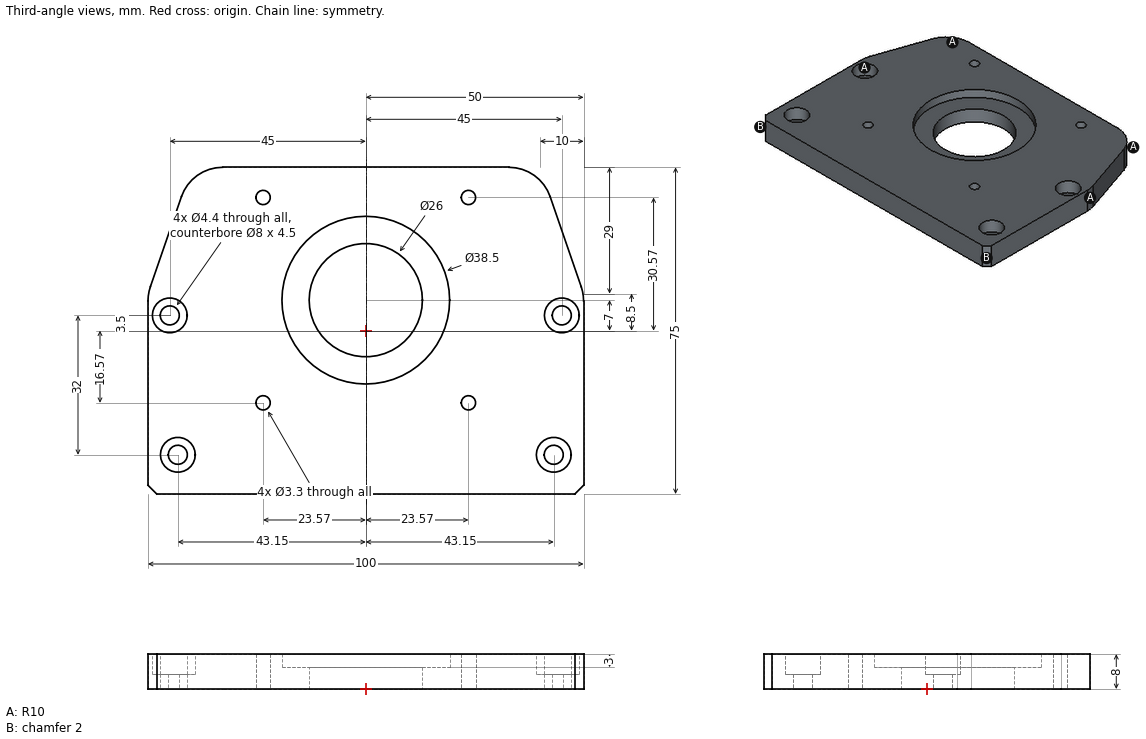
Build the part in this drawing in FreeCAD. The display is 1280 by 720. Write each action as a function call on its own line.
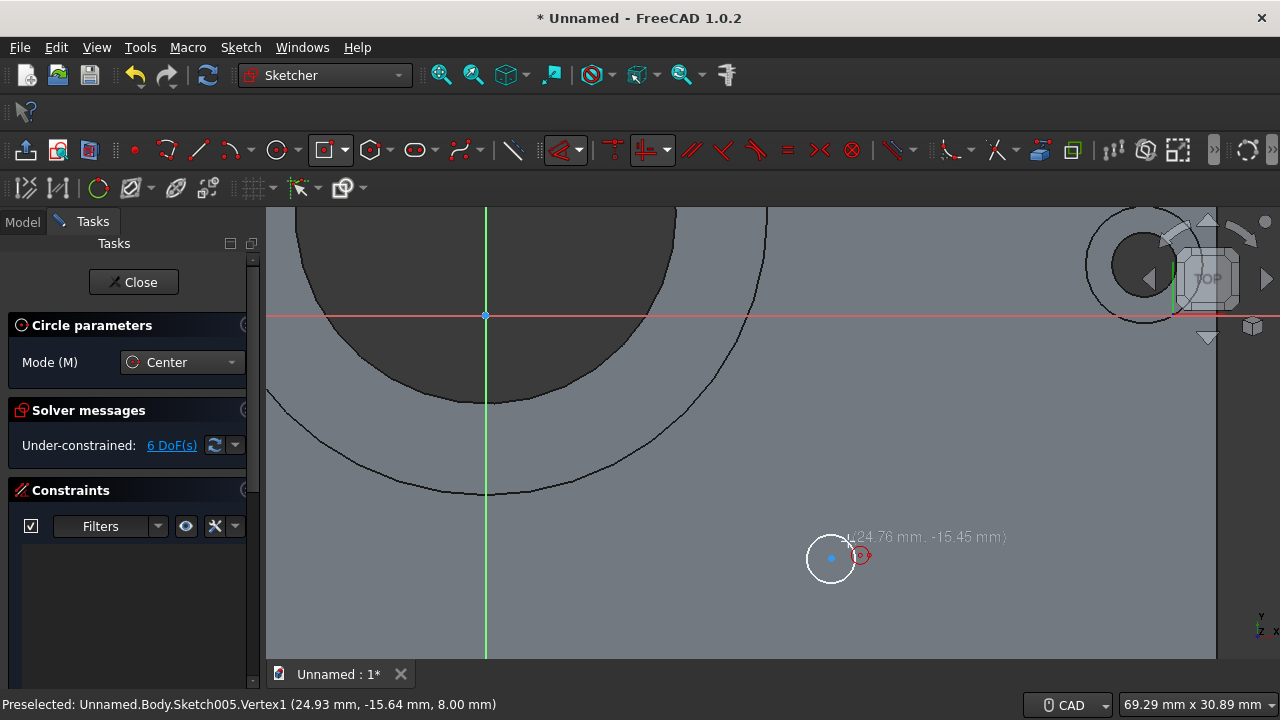
scroll(832, 561, down, 5)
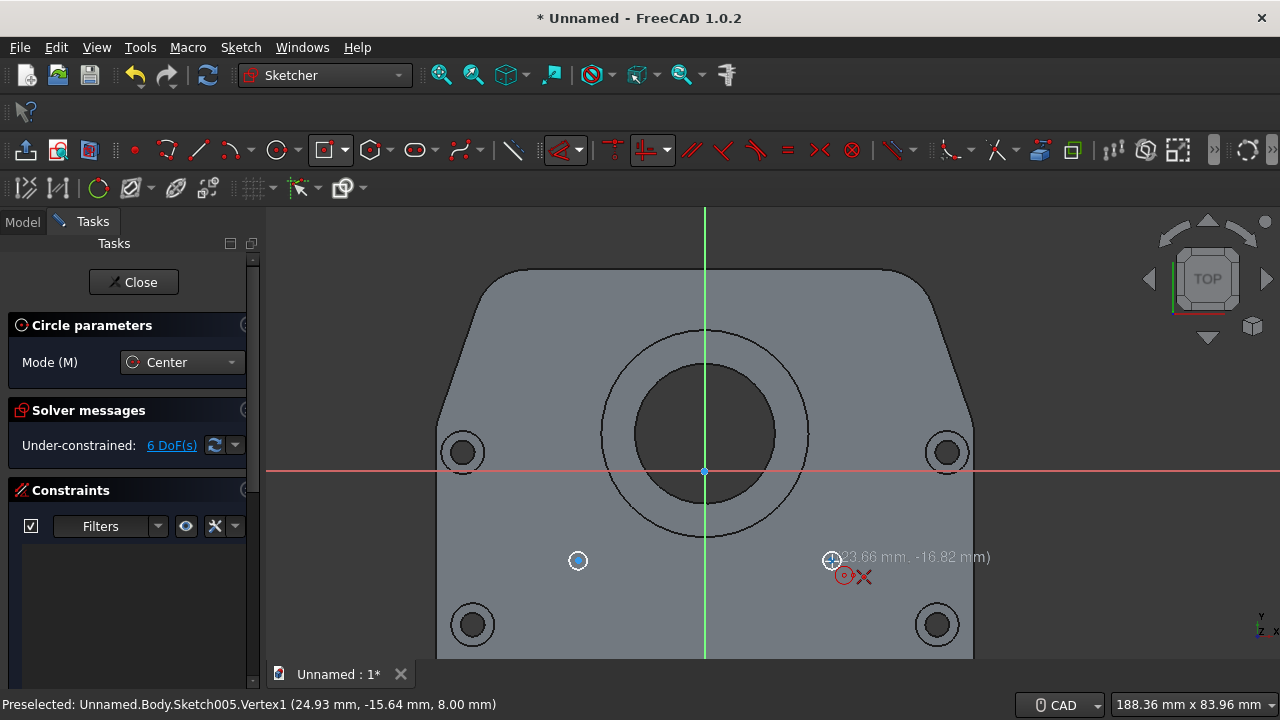
scroll(832, 307, up, 5)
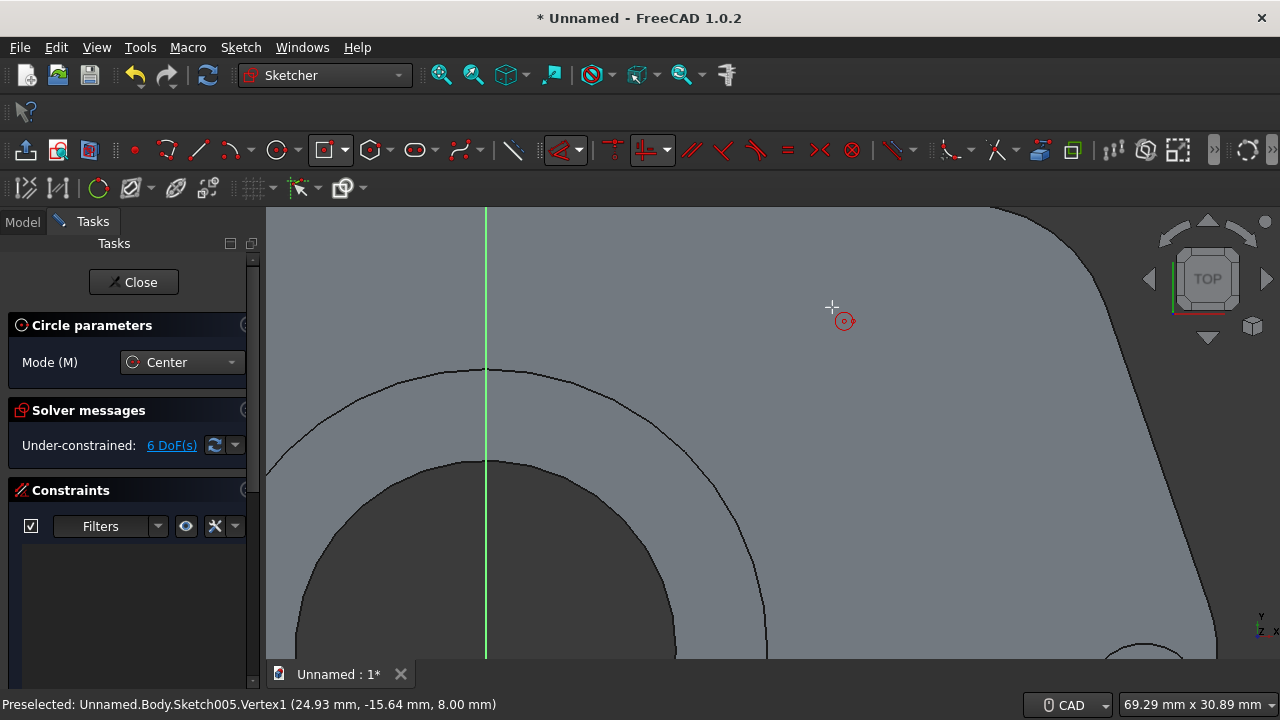
click(831, 306)
click(848, 289)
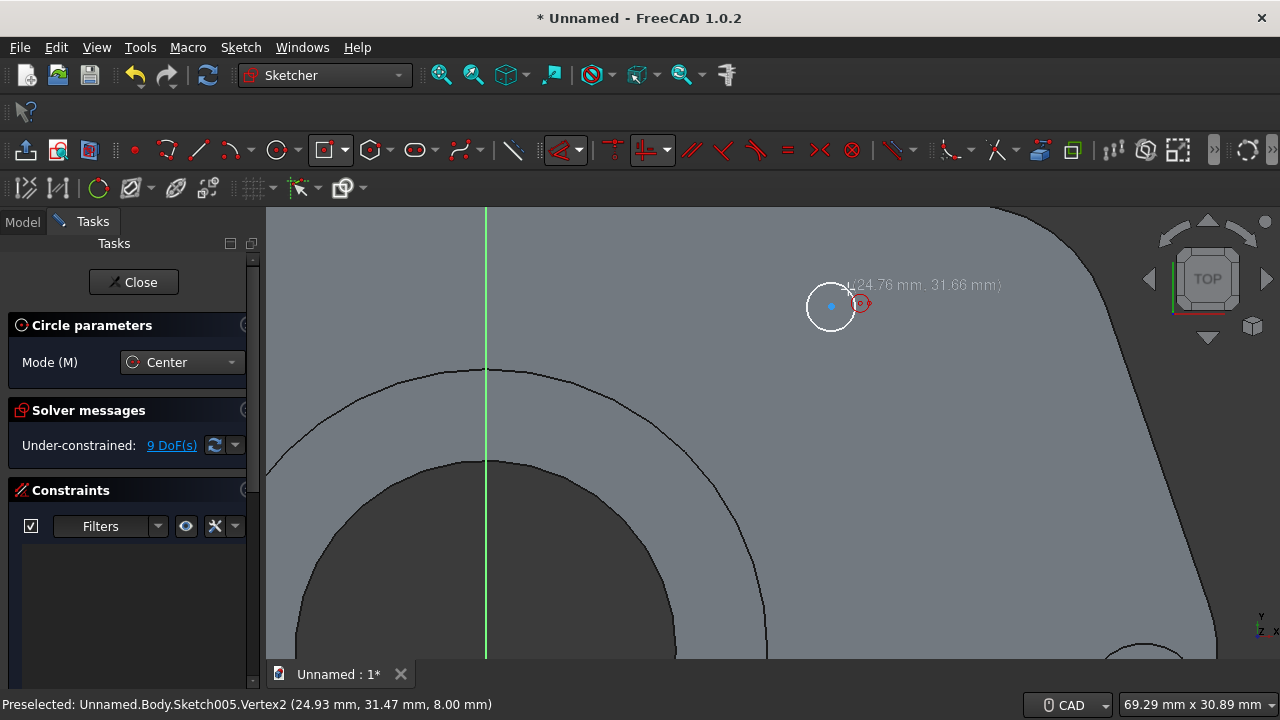
scroll(832, 306, down, 5)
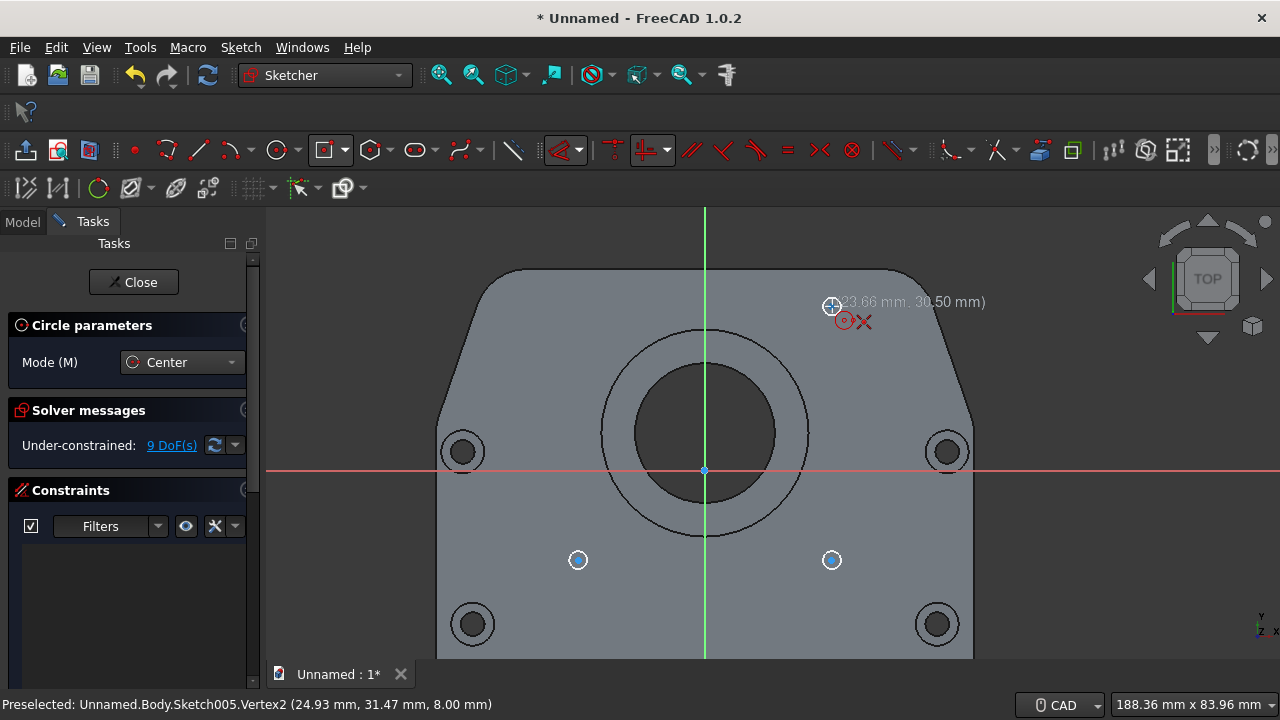
scroll(578, 306, up, 5)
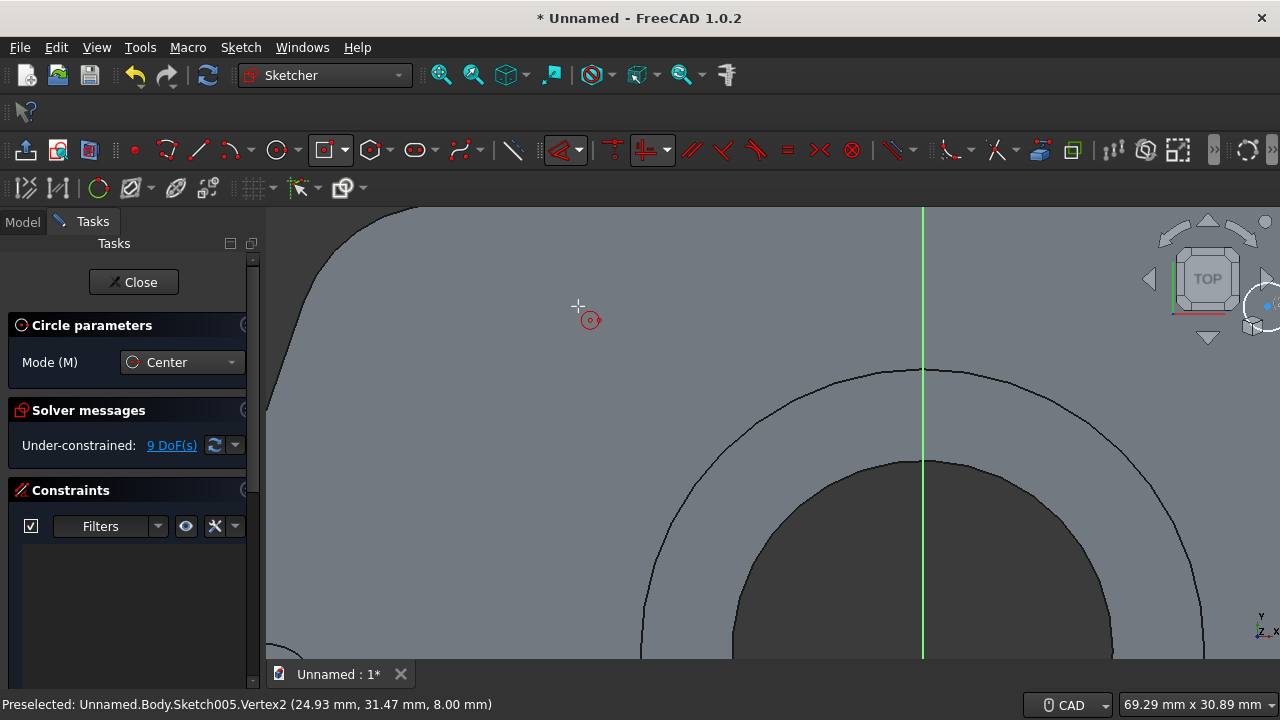
click(578, 306)
click(595, 289)
key(Escape)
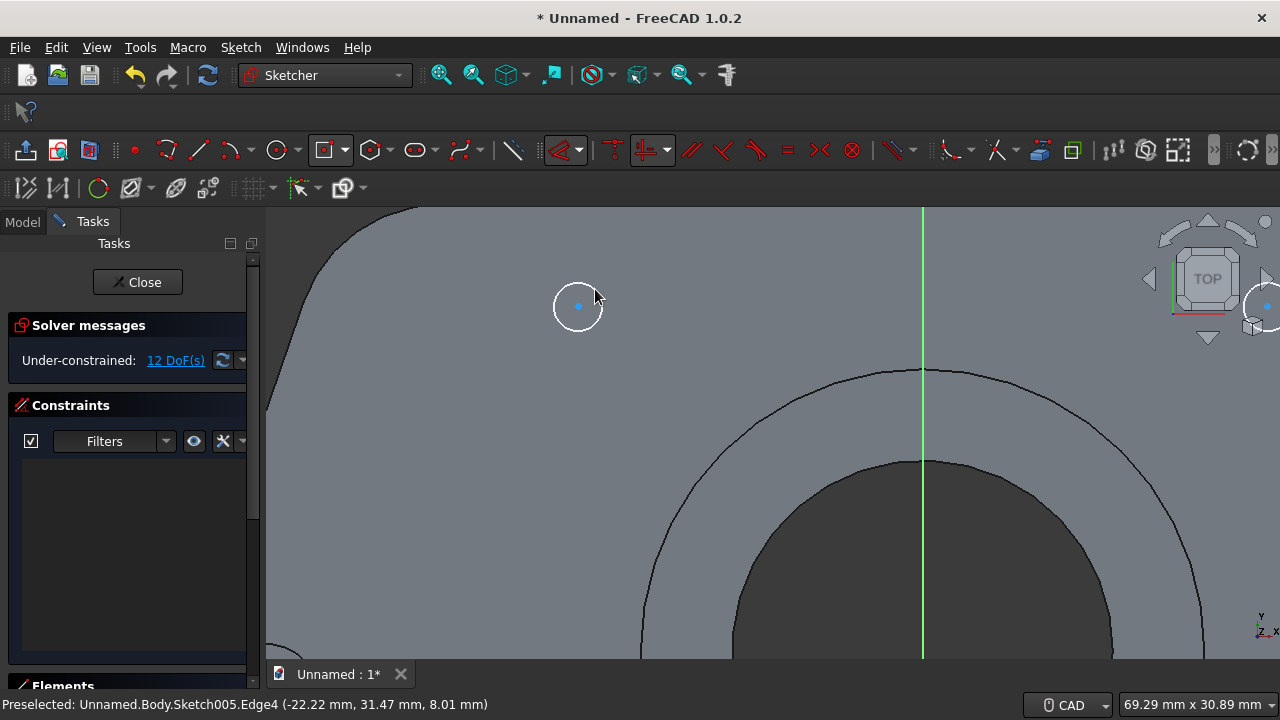
scroll(578, 306, down, 5)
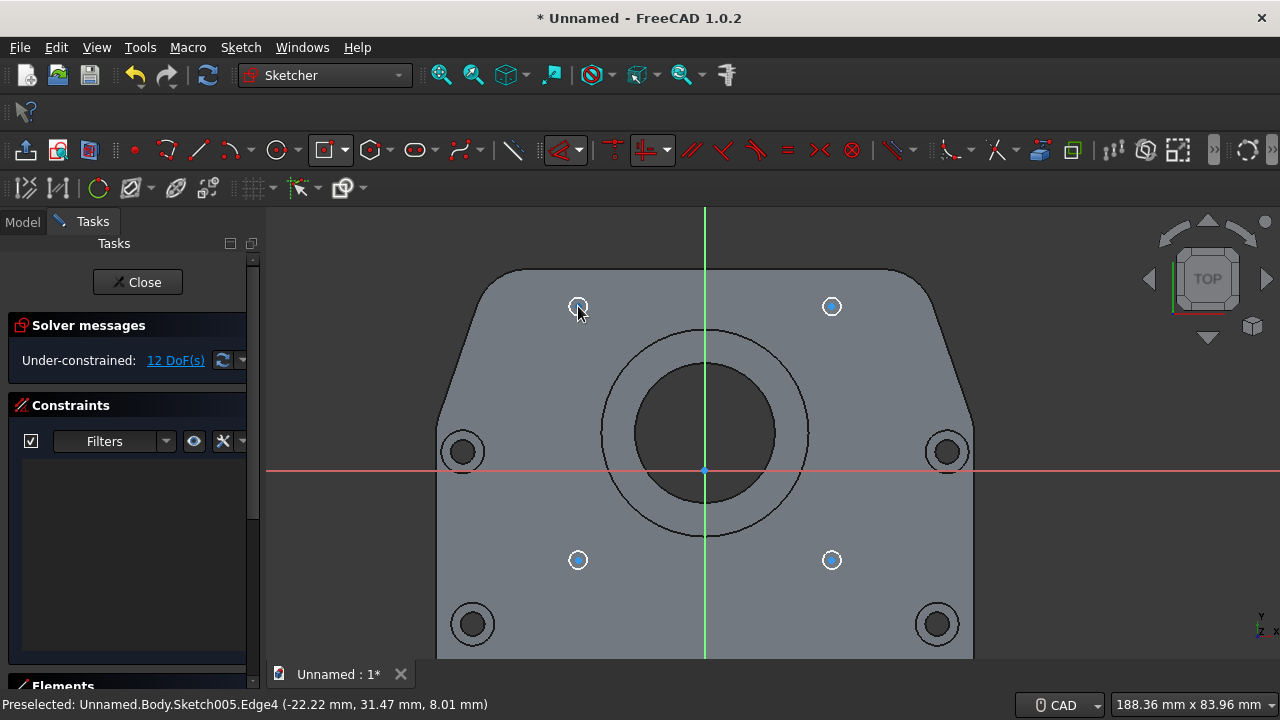
scroll(584, 554, up, 3)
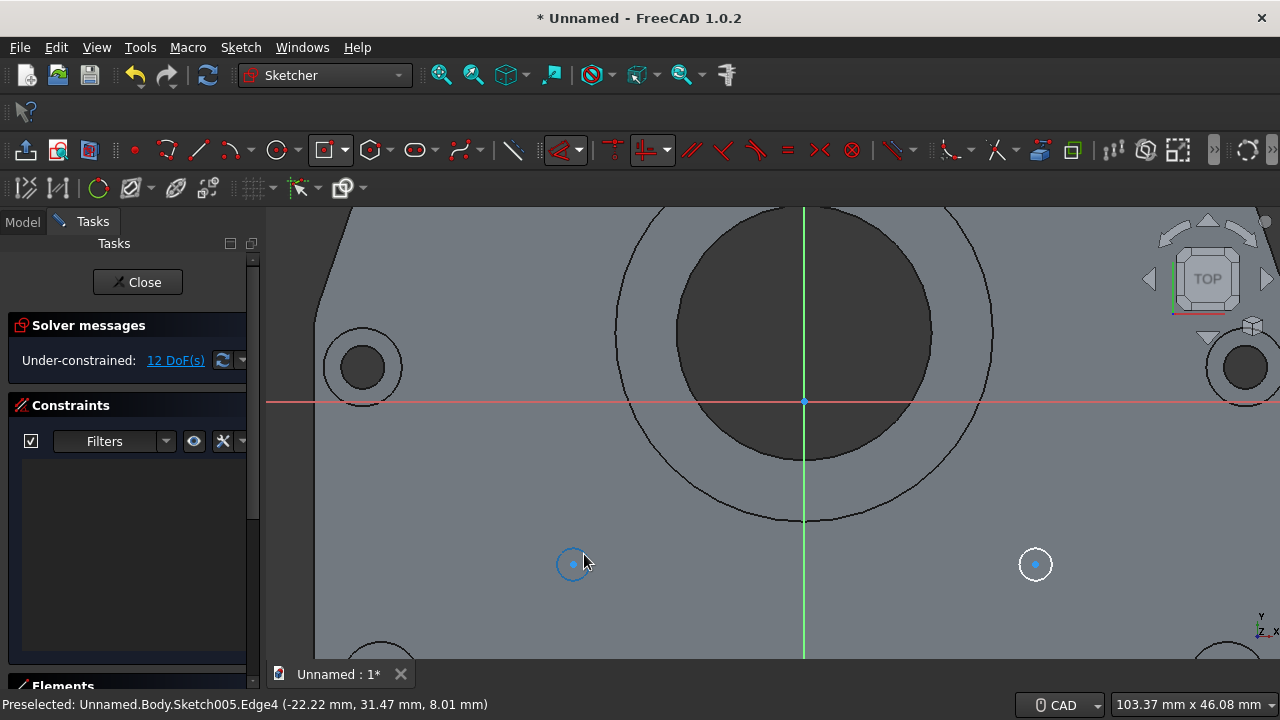
click(585, 553)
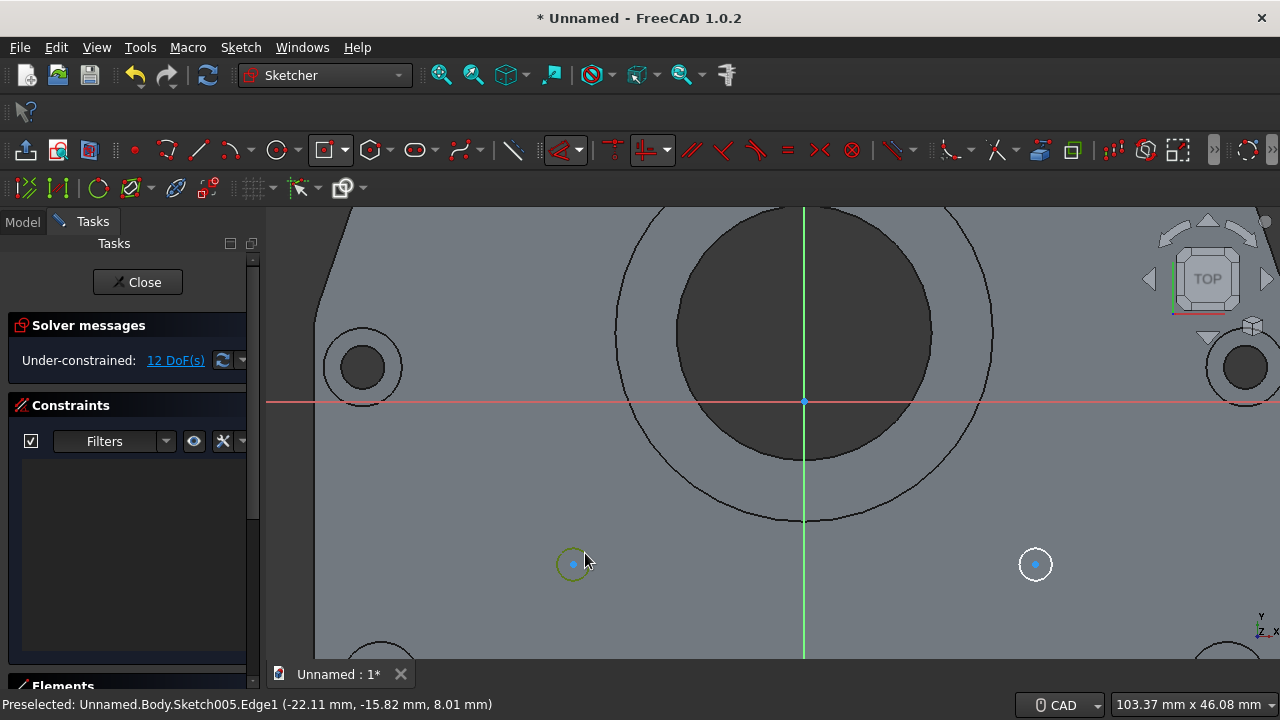
click(1047, 553)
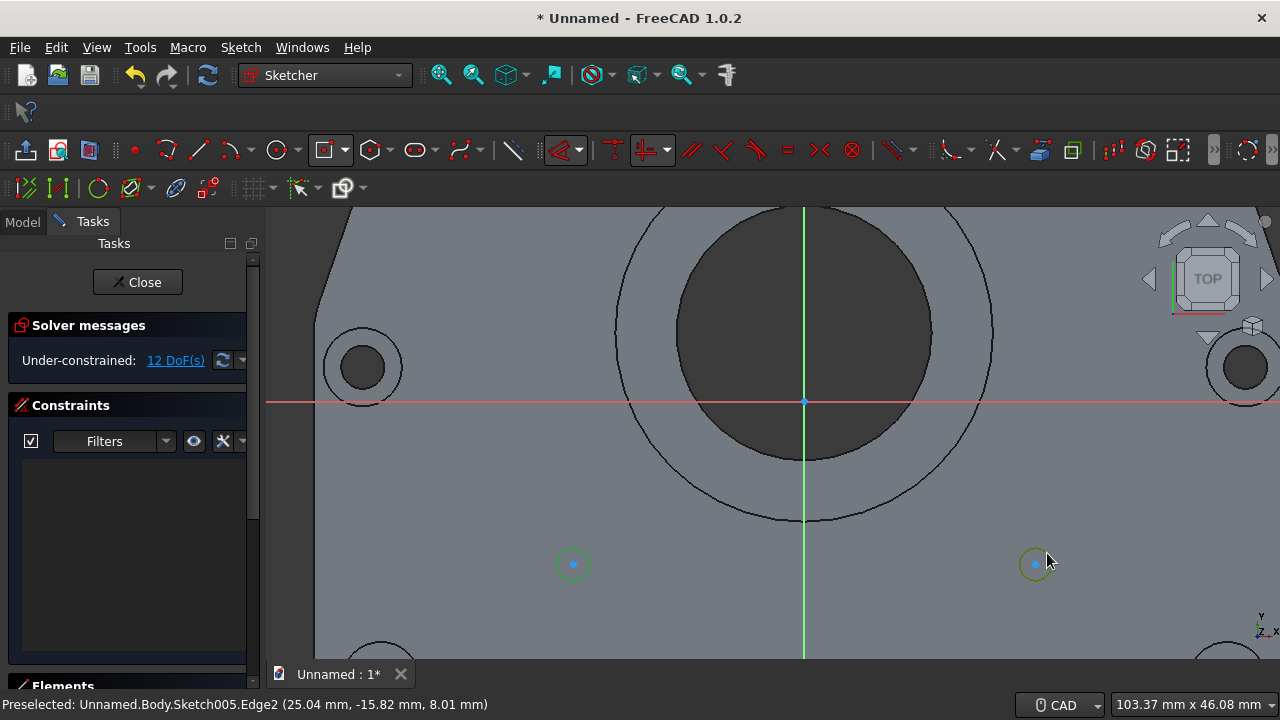
scroll(583, 555, down, 3)